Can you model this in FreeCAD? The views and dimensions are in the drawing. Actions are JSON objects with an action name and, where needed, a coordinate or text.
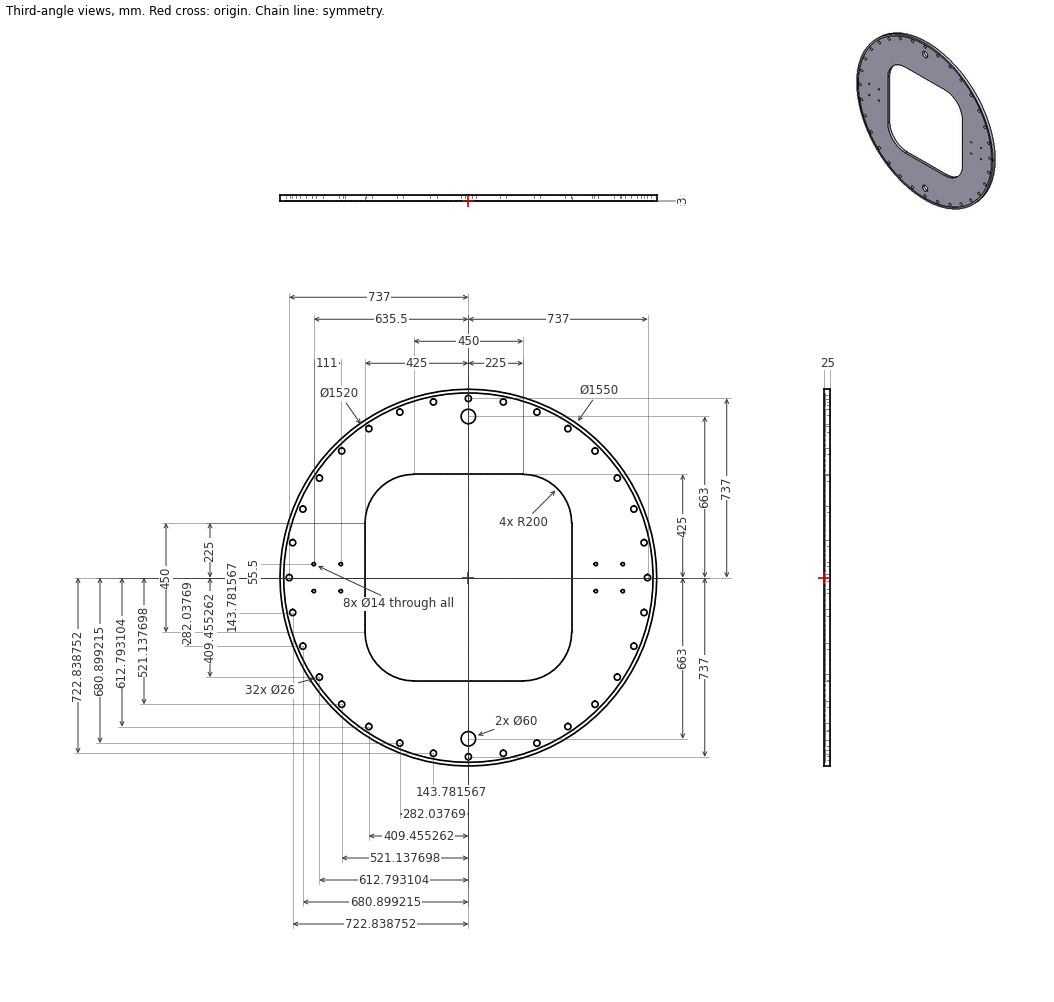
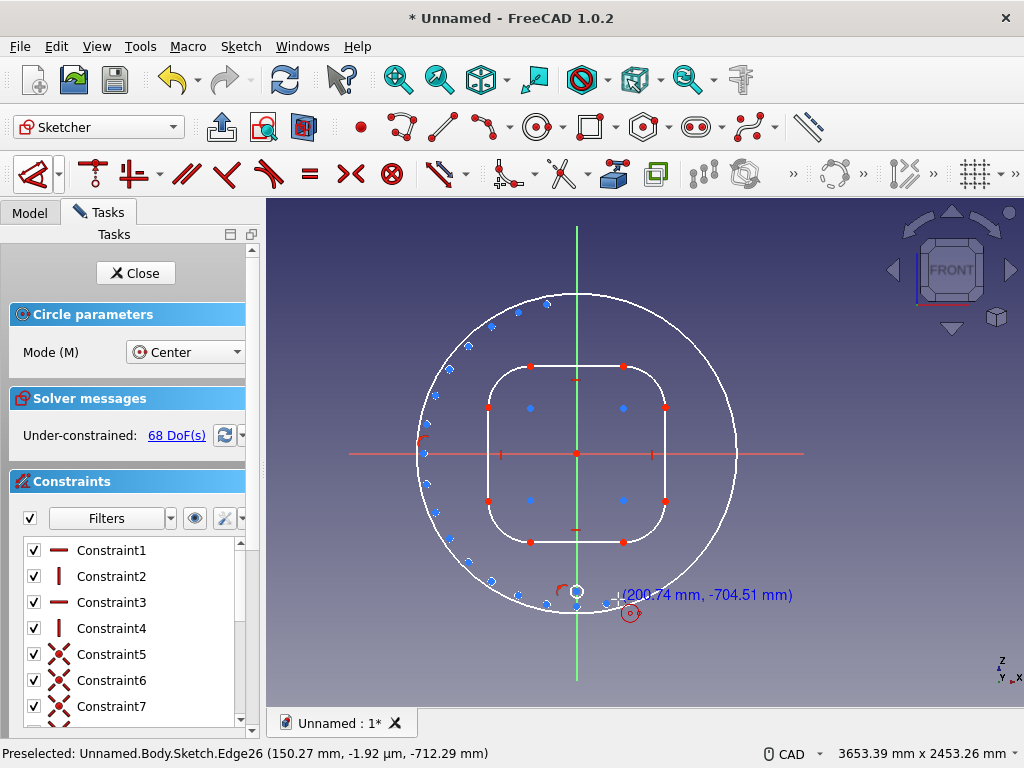
{"action": "scroll", "coordinate": [635, 595], "scroll_direction": "up", "scroll_amount": 4}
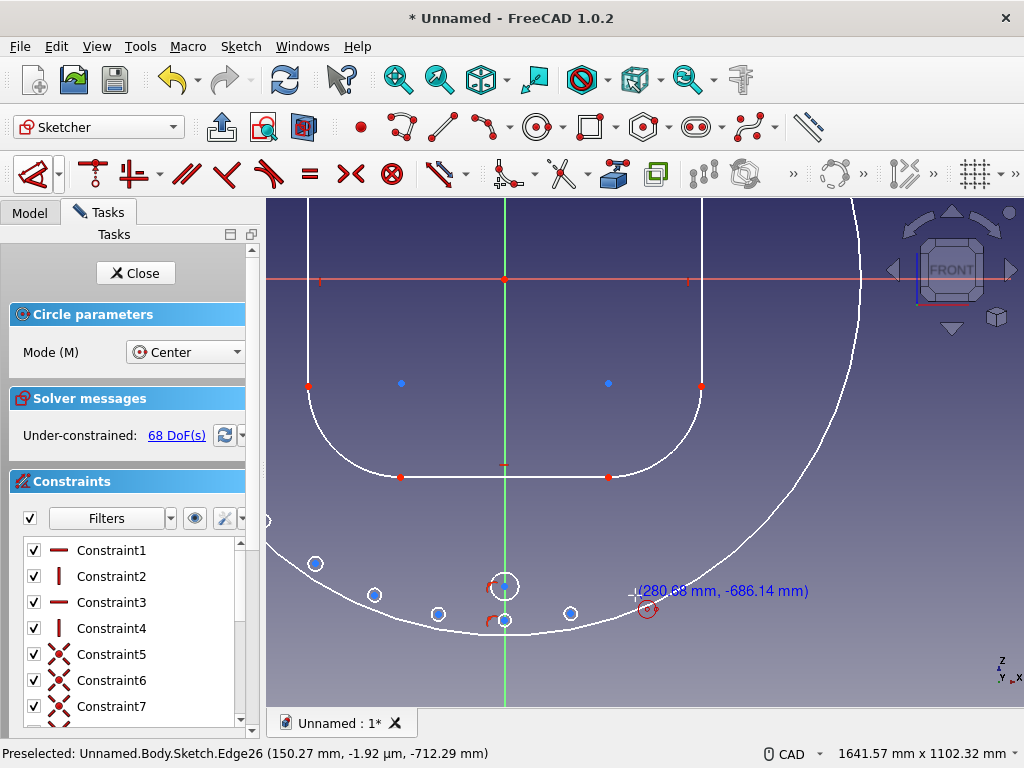
{"action": "left_click", "coordinate": [635, 594]}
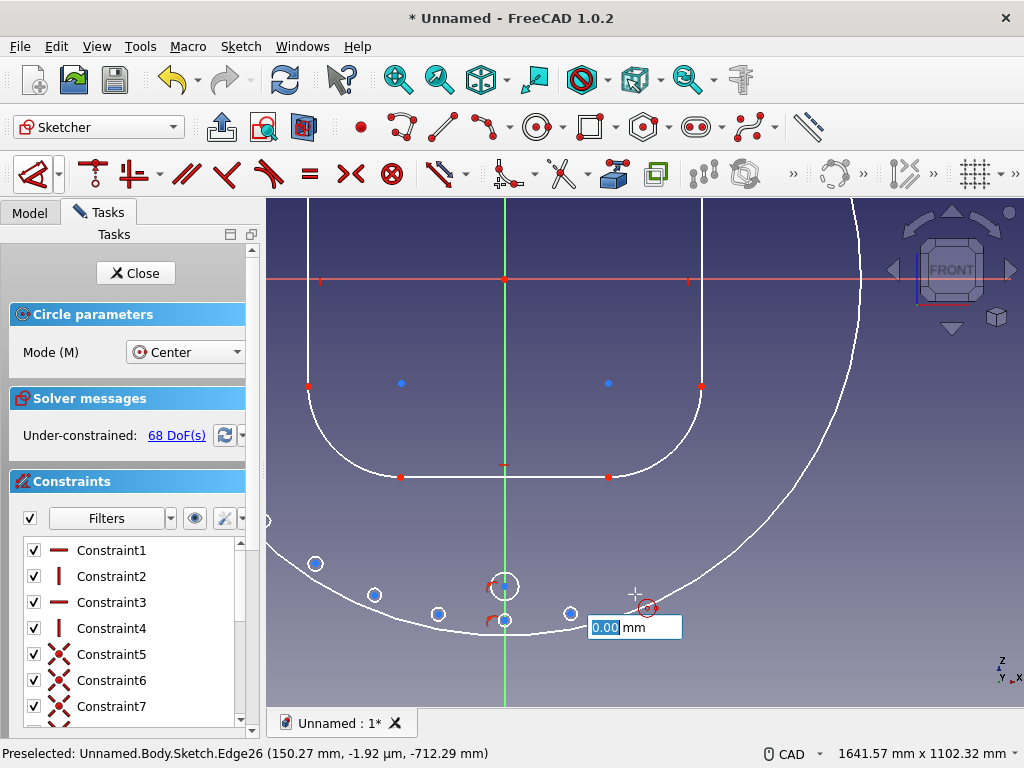
{"action": "scroll", "coordinate": [639, 590], "scroll_direction": "up", "scroll_amount": 5}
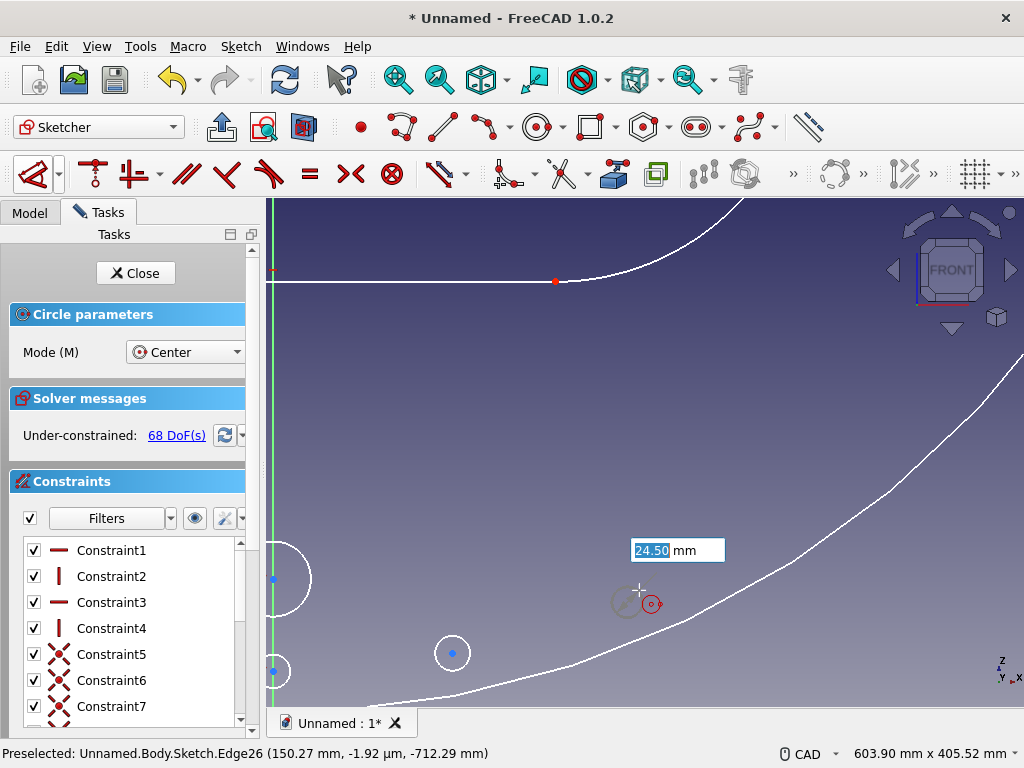
{"action": "left_click", "coordinate": [639, 588]}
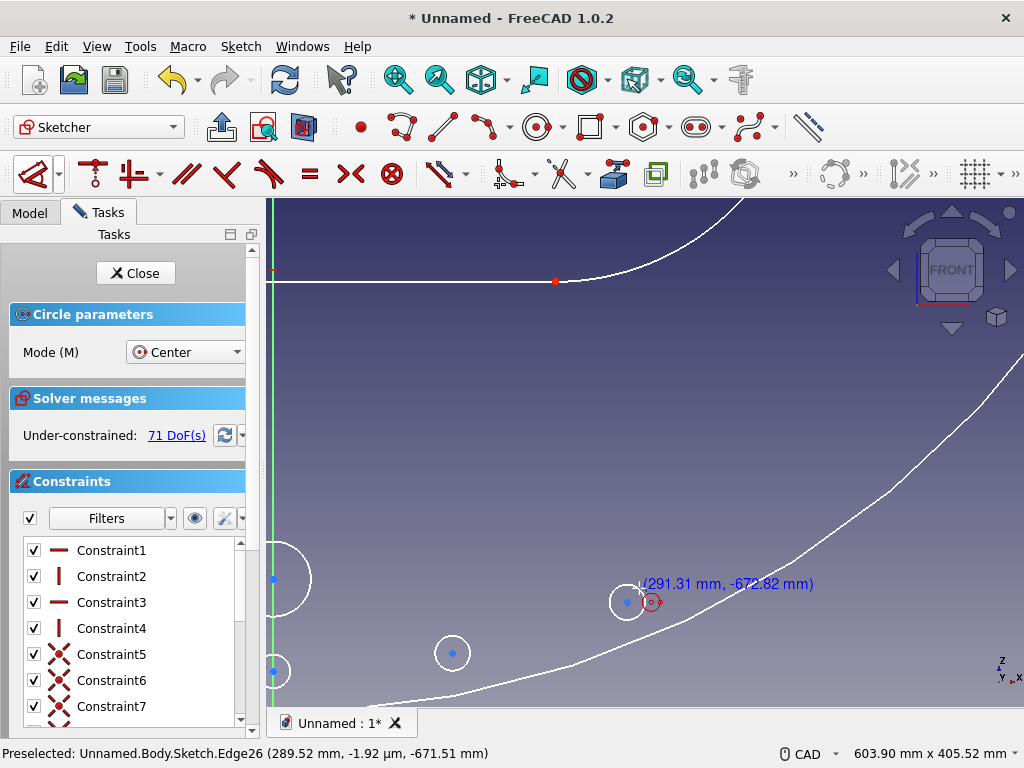
{"action": "scroll", "coordinate": [787, 514], "scroll_direction": "up", "scroll_amount": 2}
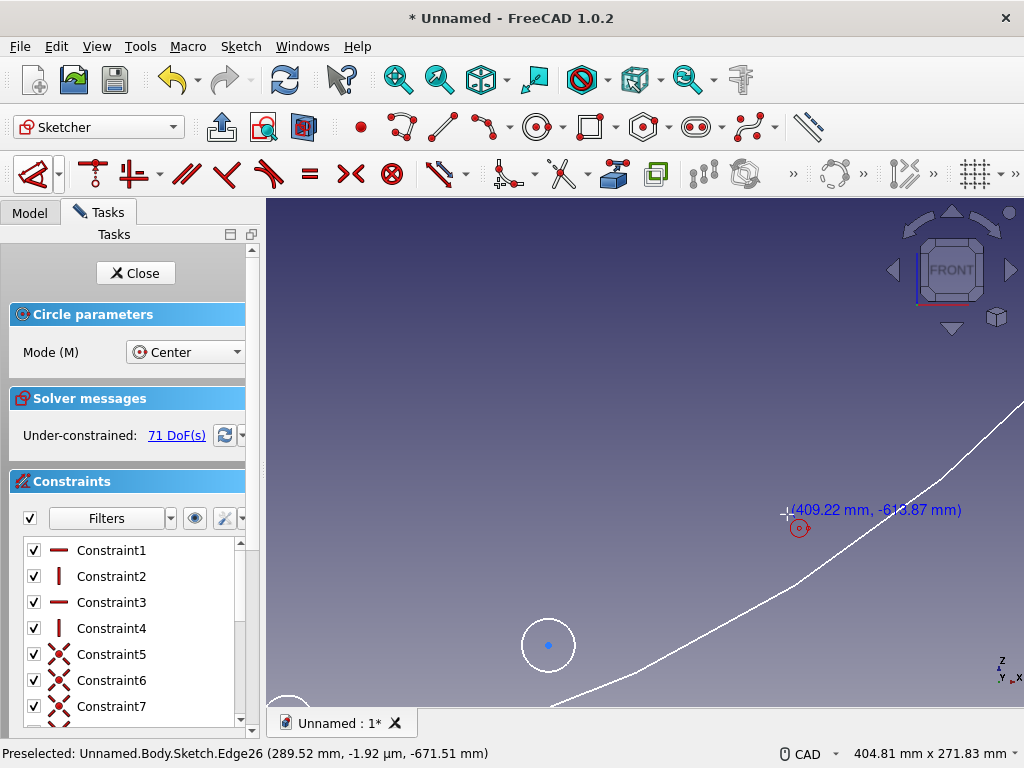
{"action": "scroll", "coordinate": [646, 588], "scroll_direction": "down", "scroll_amount": 11}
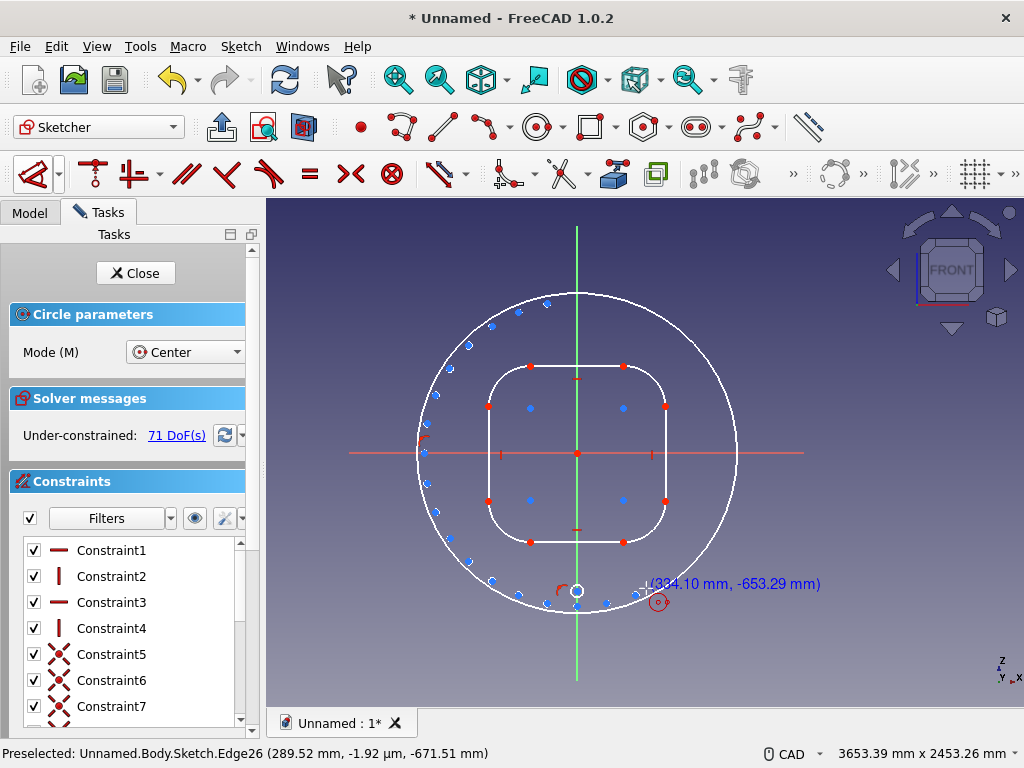
{"action": "scroll", "coordinate": [662, 580], "scroll_direction": "up", "scroll_amount": 4}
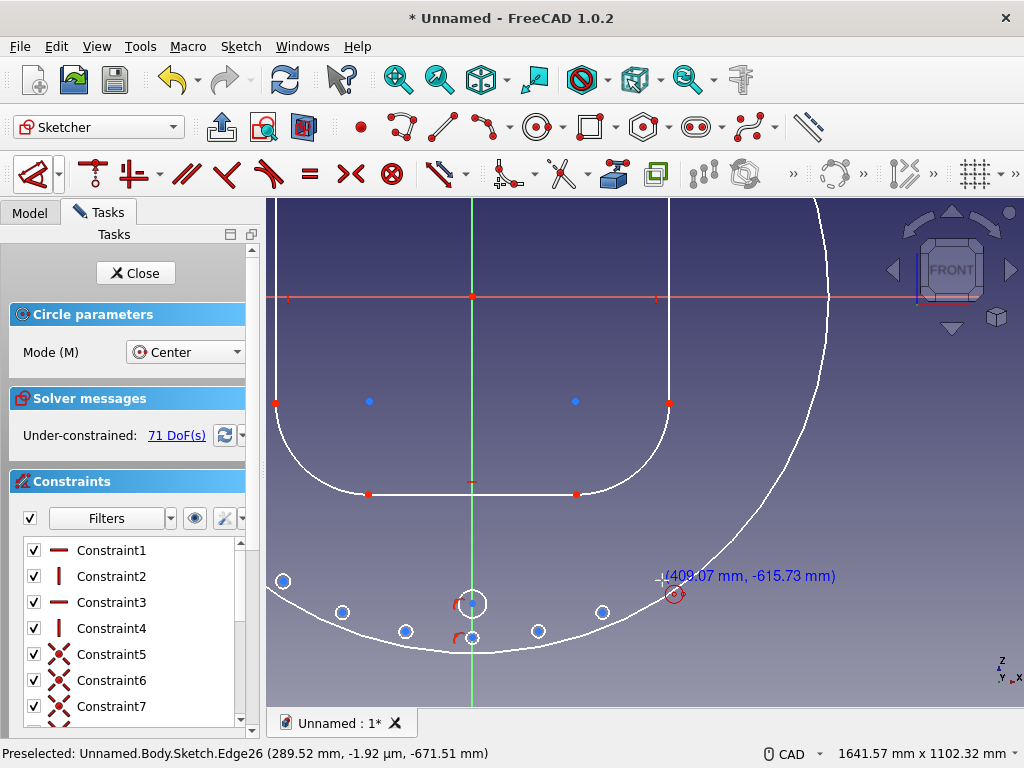
{"action": "left_click", "coordinate": [662, 580]}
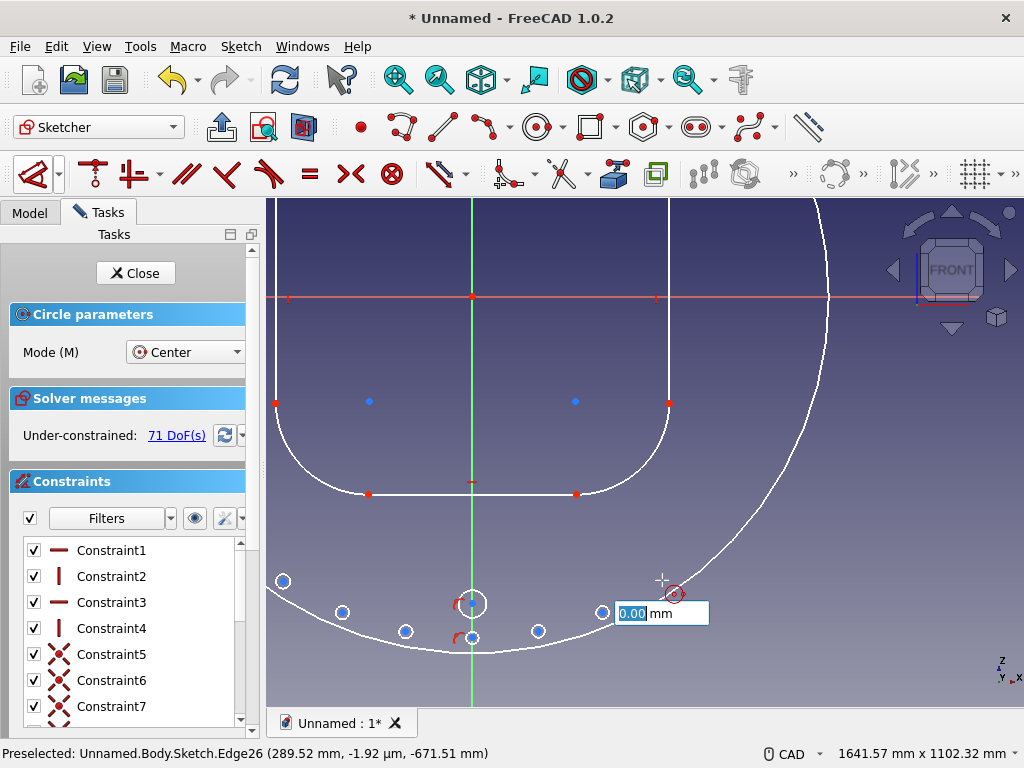
{"action": "scroll", "coordinate": [666, 576], "scroll_direction": "up", "scroll_amount": 5}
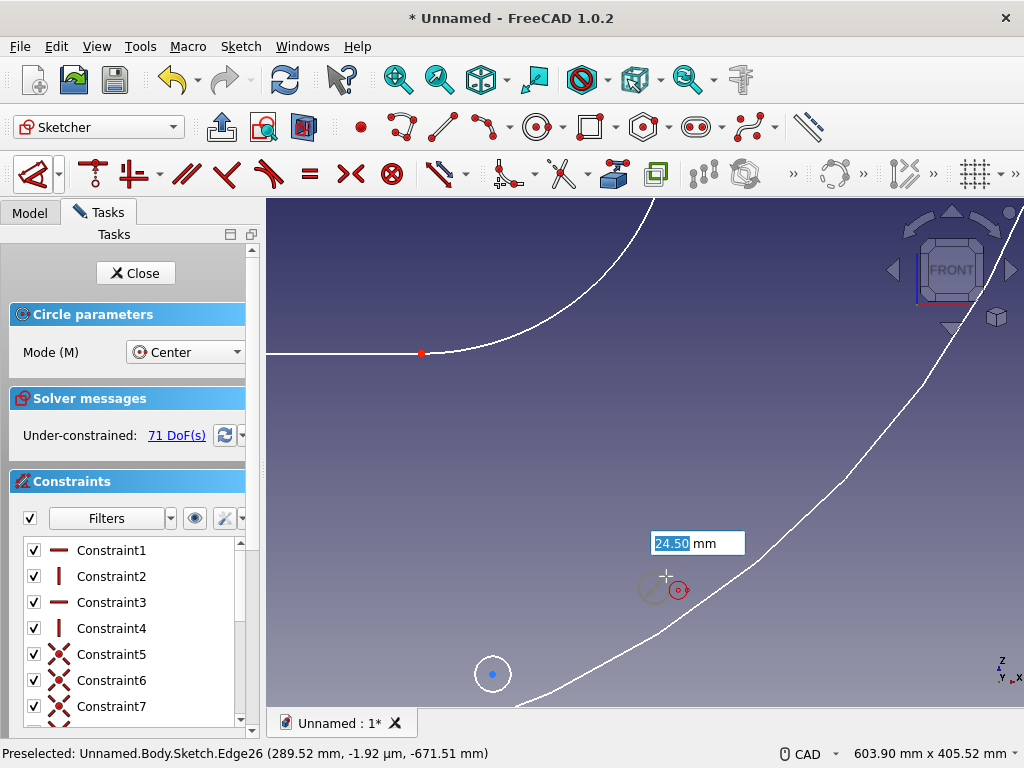
{"action": "left_click", "coordinate": [664, 574]}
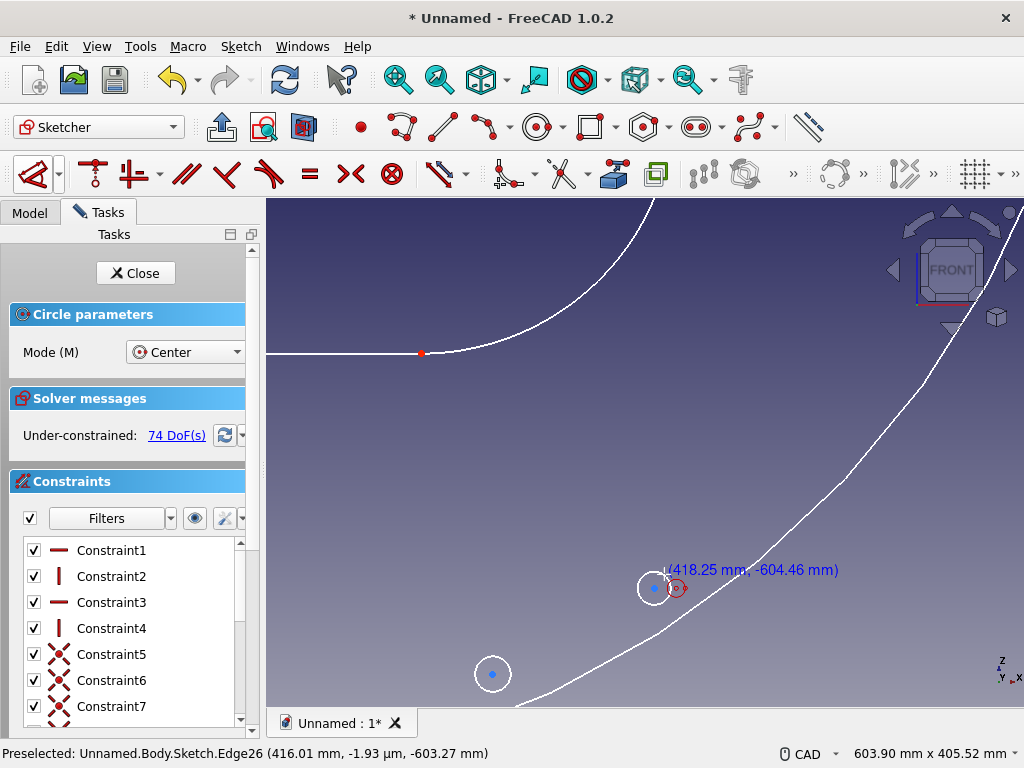
{"action": "scroll", "coordinate": [793, 470], "scroll_direction": "up", "scroll_amount": 2}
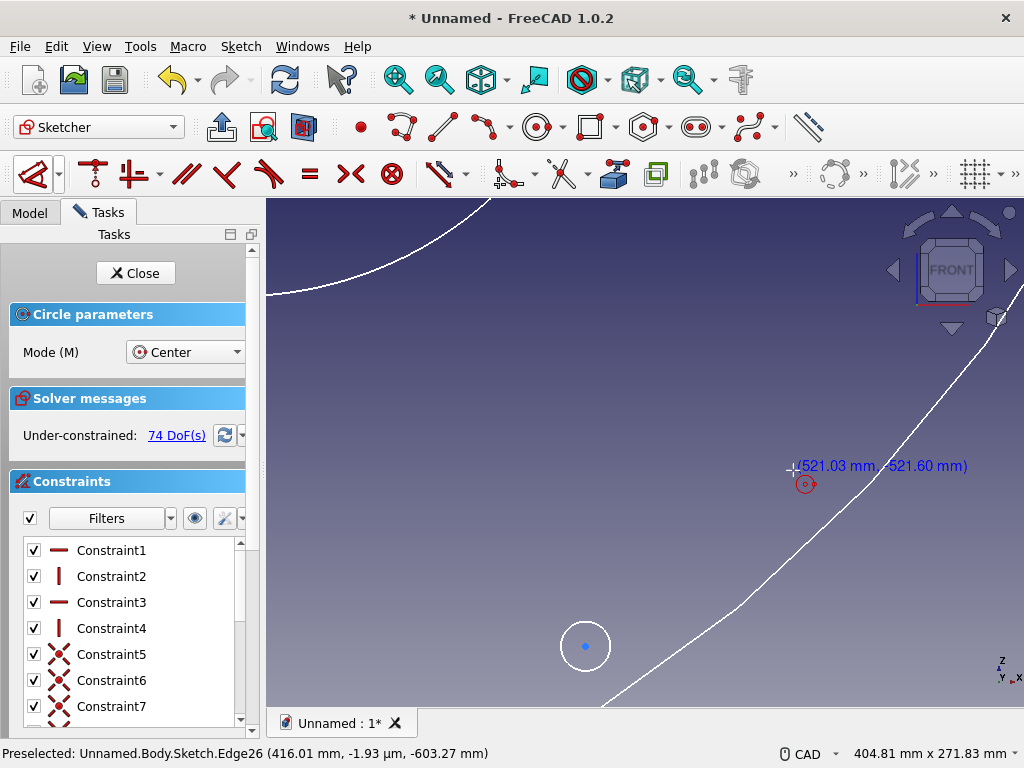
{"action": "scroll", "coordinate": [671, 572], "scroll_direction": "down", "scroll_amount": 11}